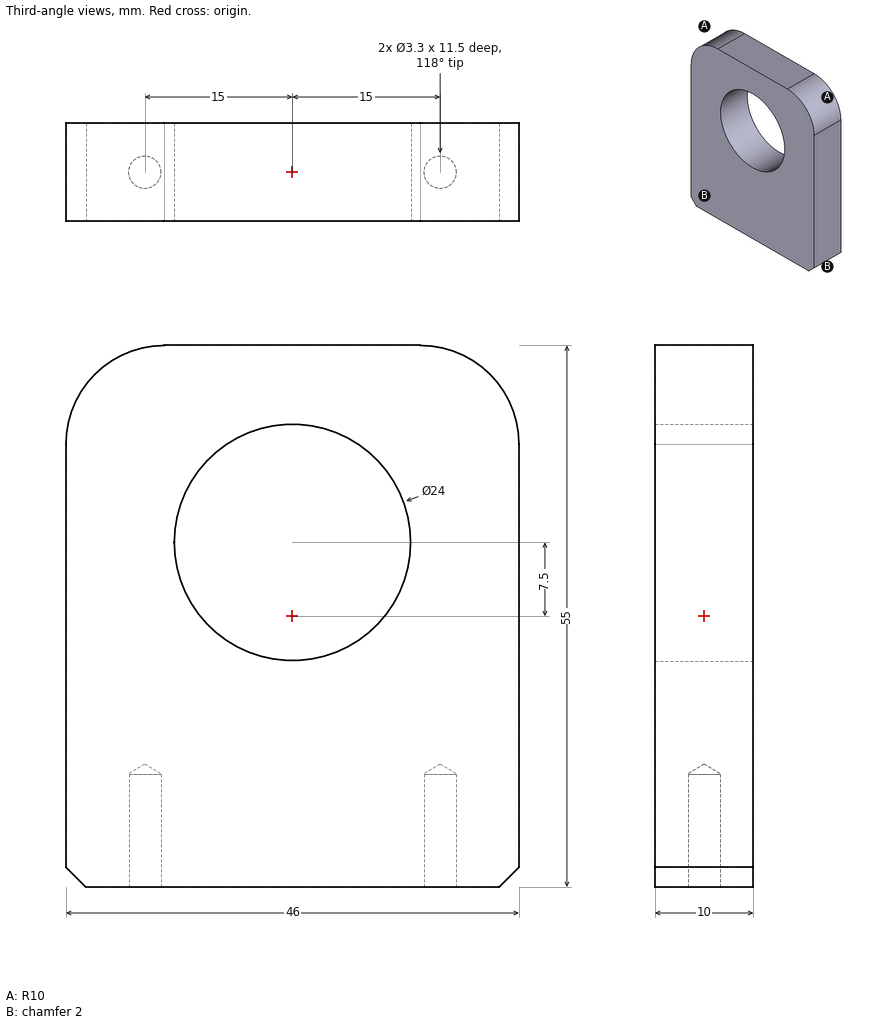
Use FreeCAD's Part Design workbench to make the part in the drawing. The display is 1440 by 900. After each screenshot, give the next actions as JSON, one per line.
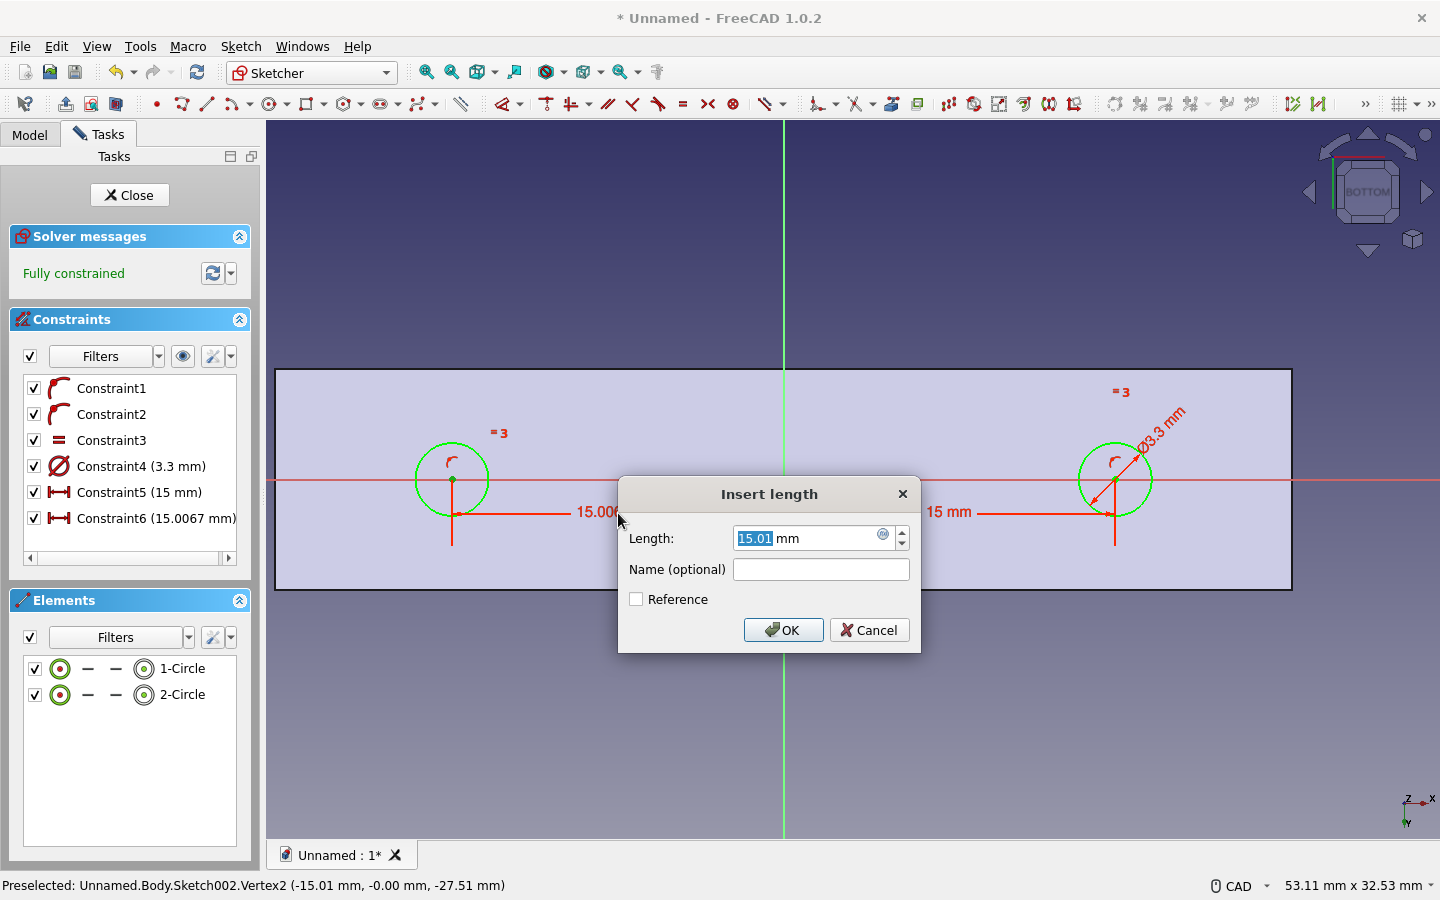
{"action": "type", "text": "15"}
{"action": "key", "text": "Return"}
{"action": "key", "text": "Escape"}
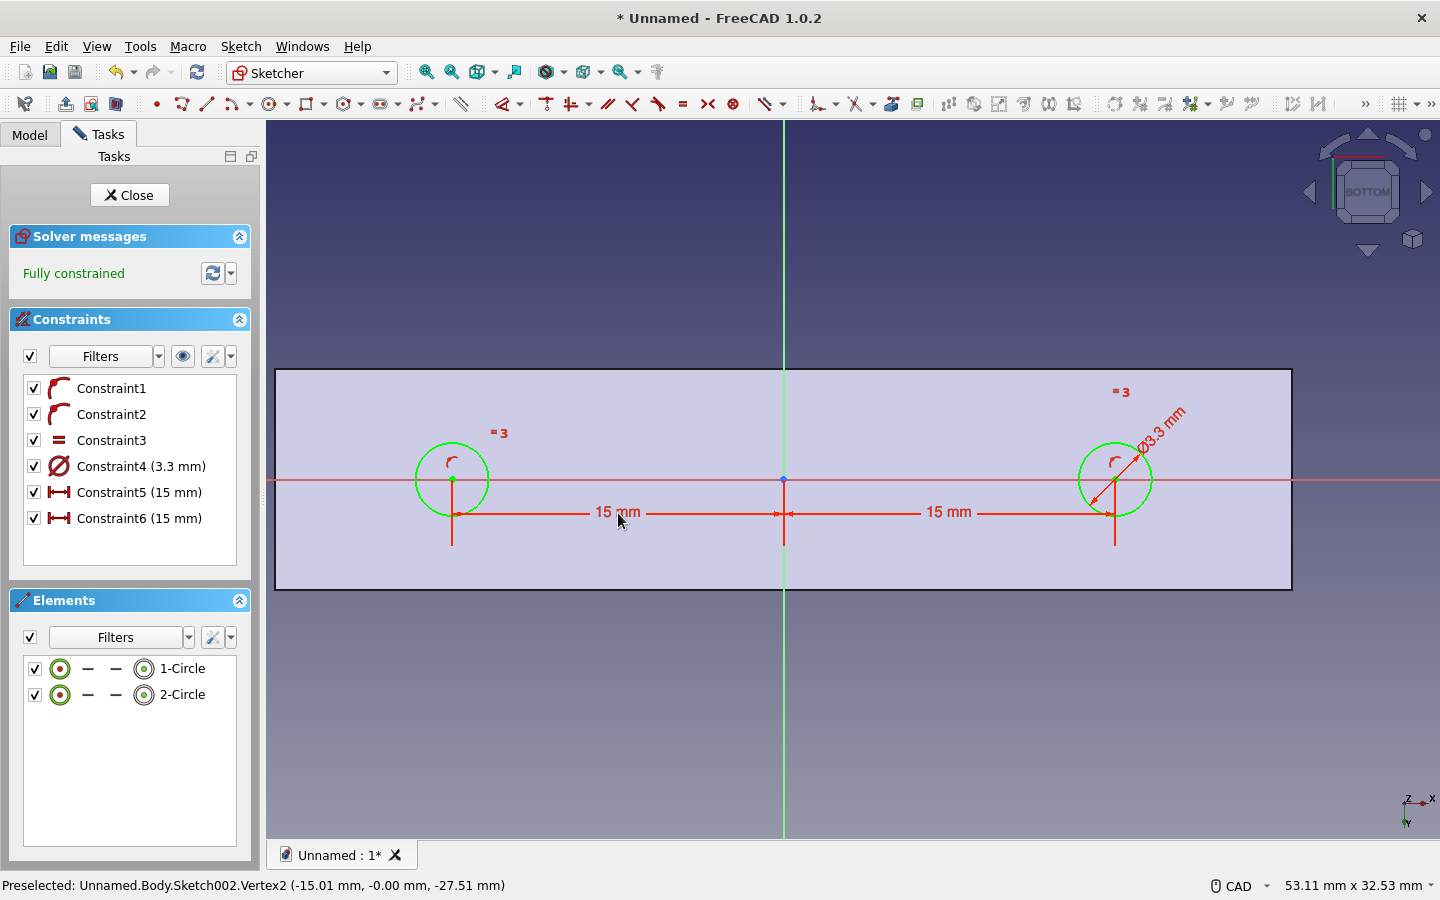
{"action": "left_click", "coordinate": [130, 195]}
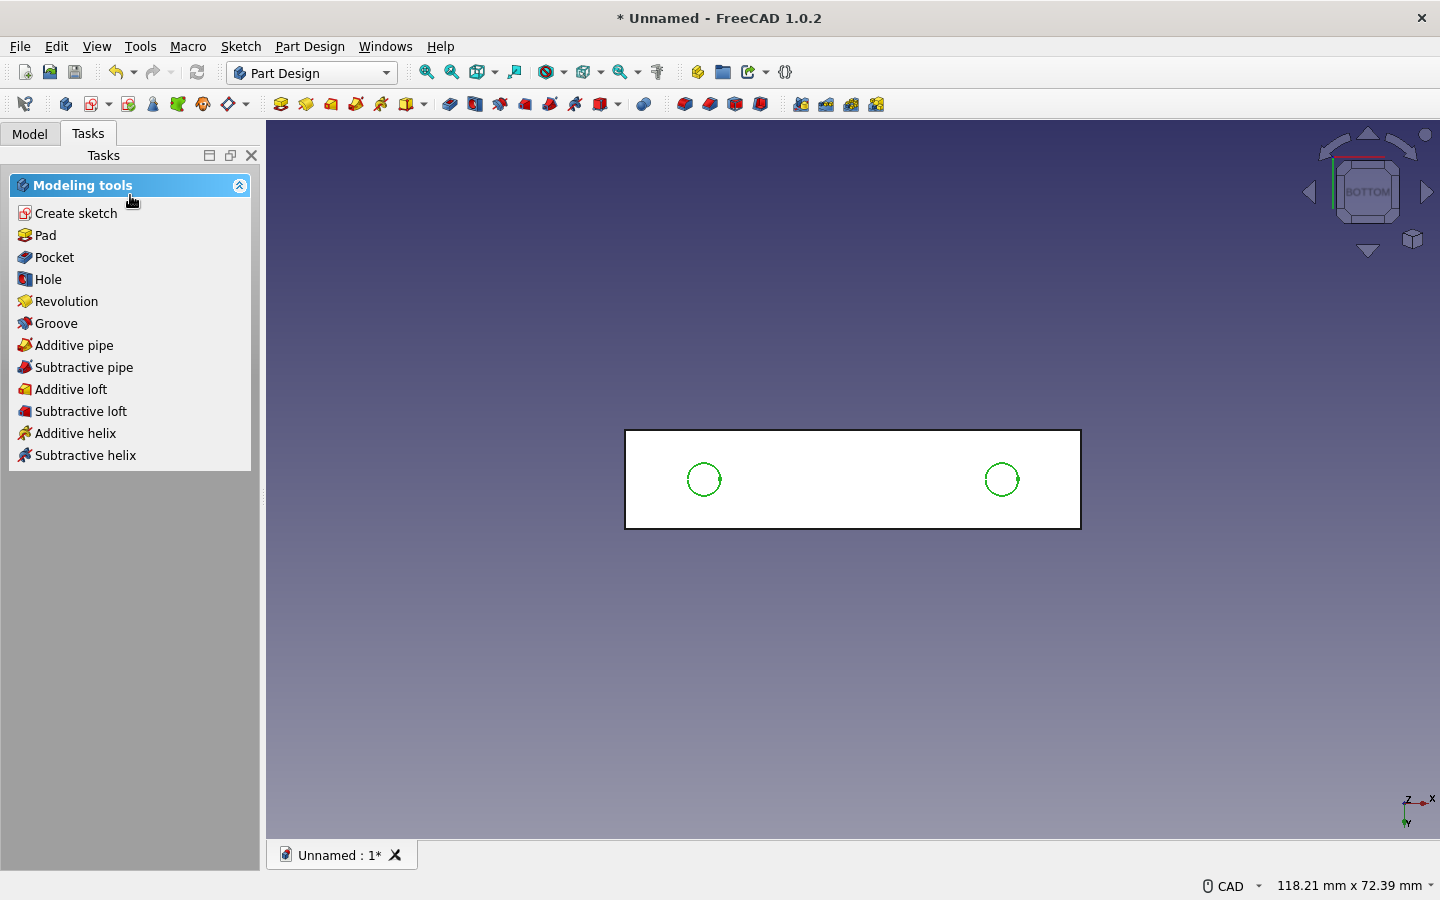
{"action": "left_click", "coordinate": [475, 104]}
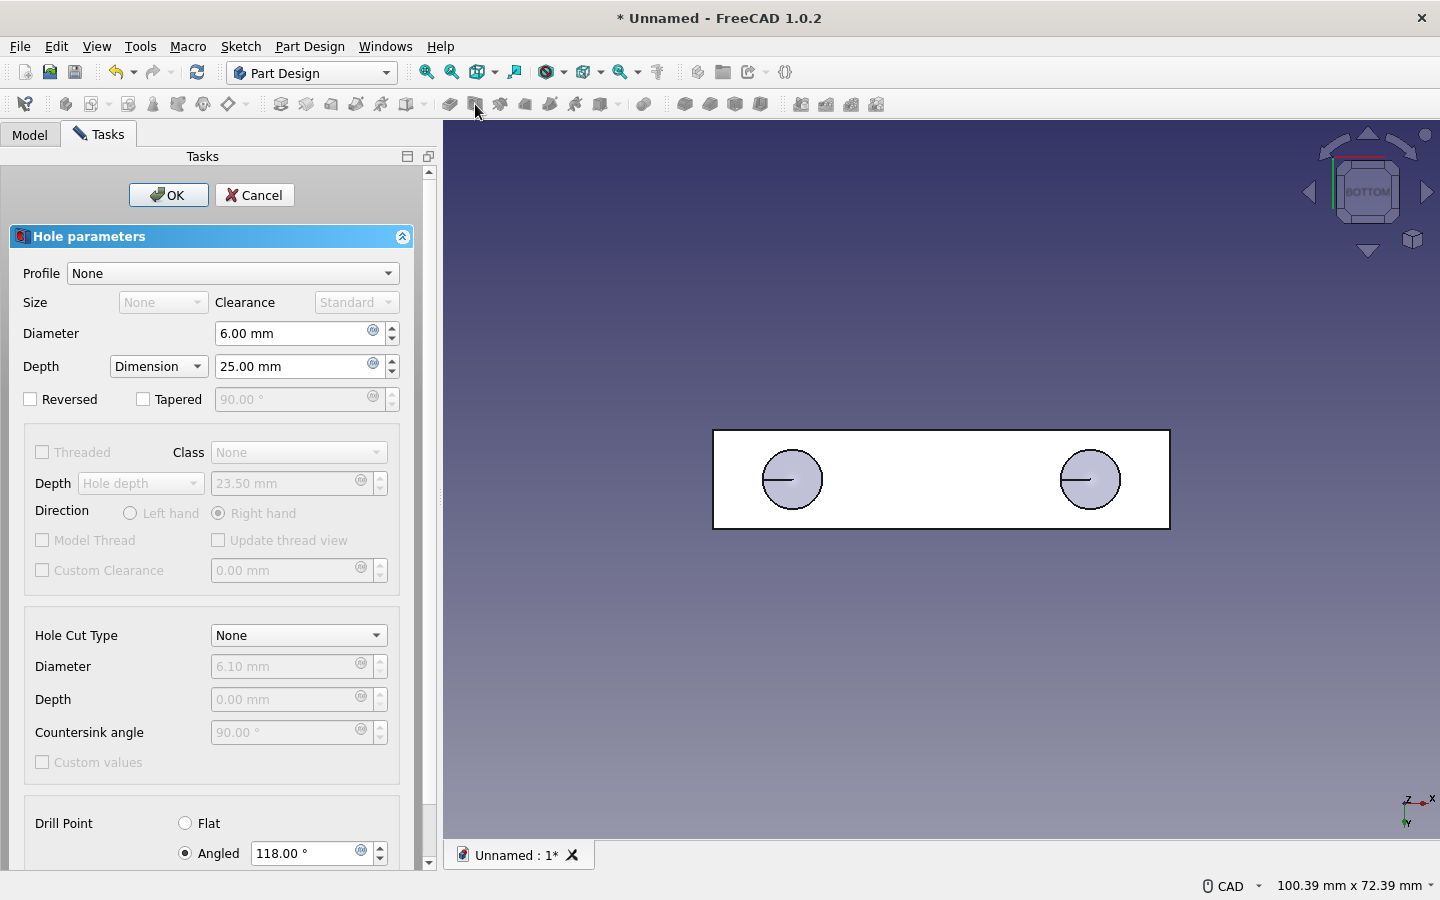
{"action": "triple_click", "coordinate": [300, 334]}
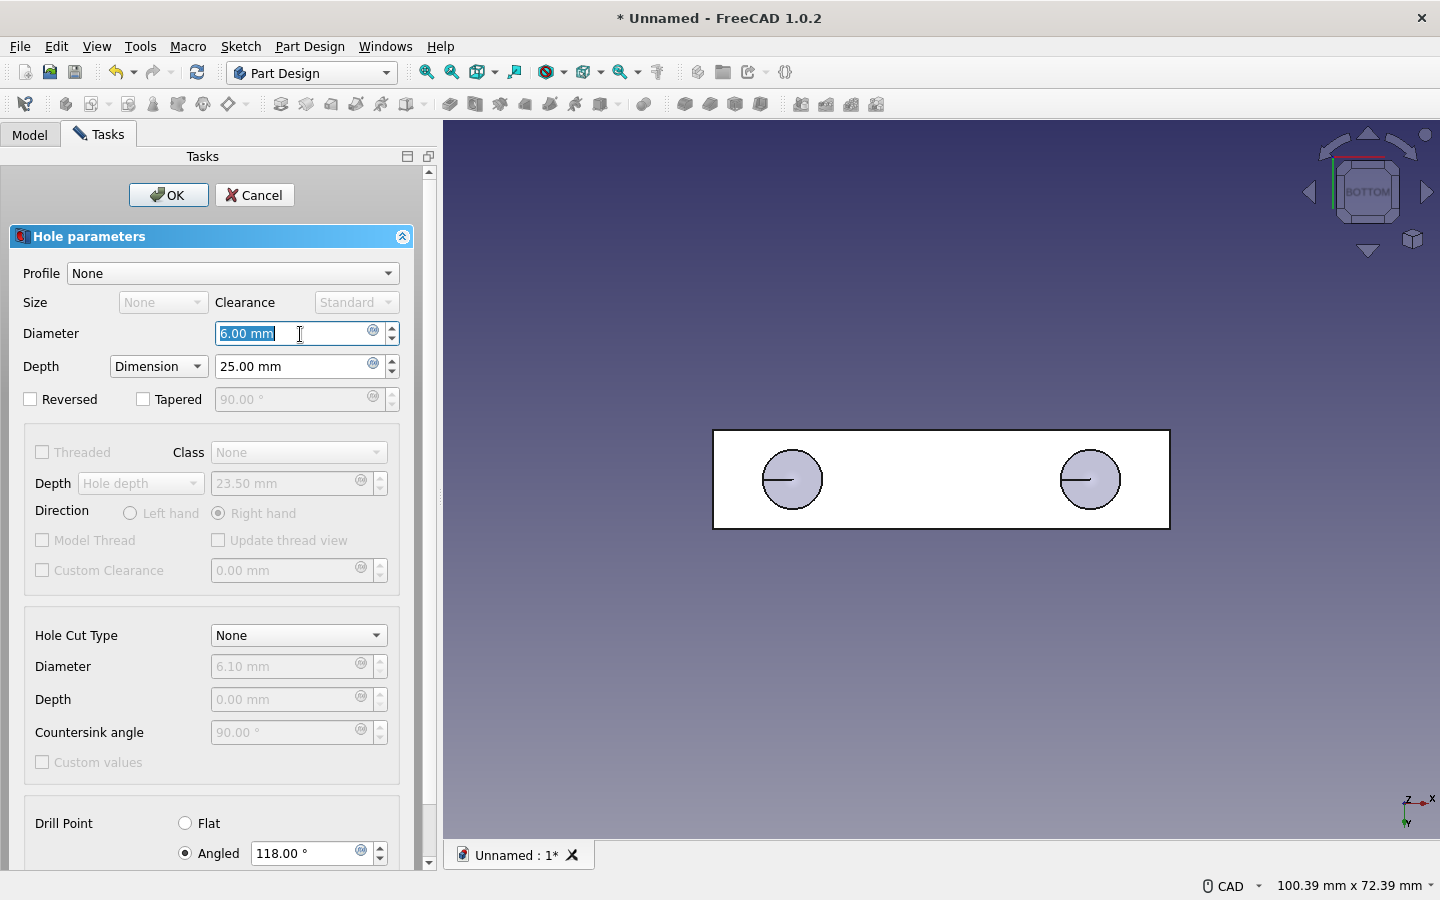
{"action": "type", "text": "3.3"}
{"action": "key", "text": "Tab"}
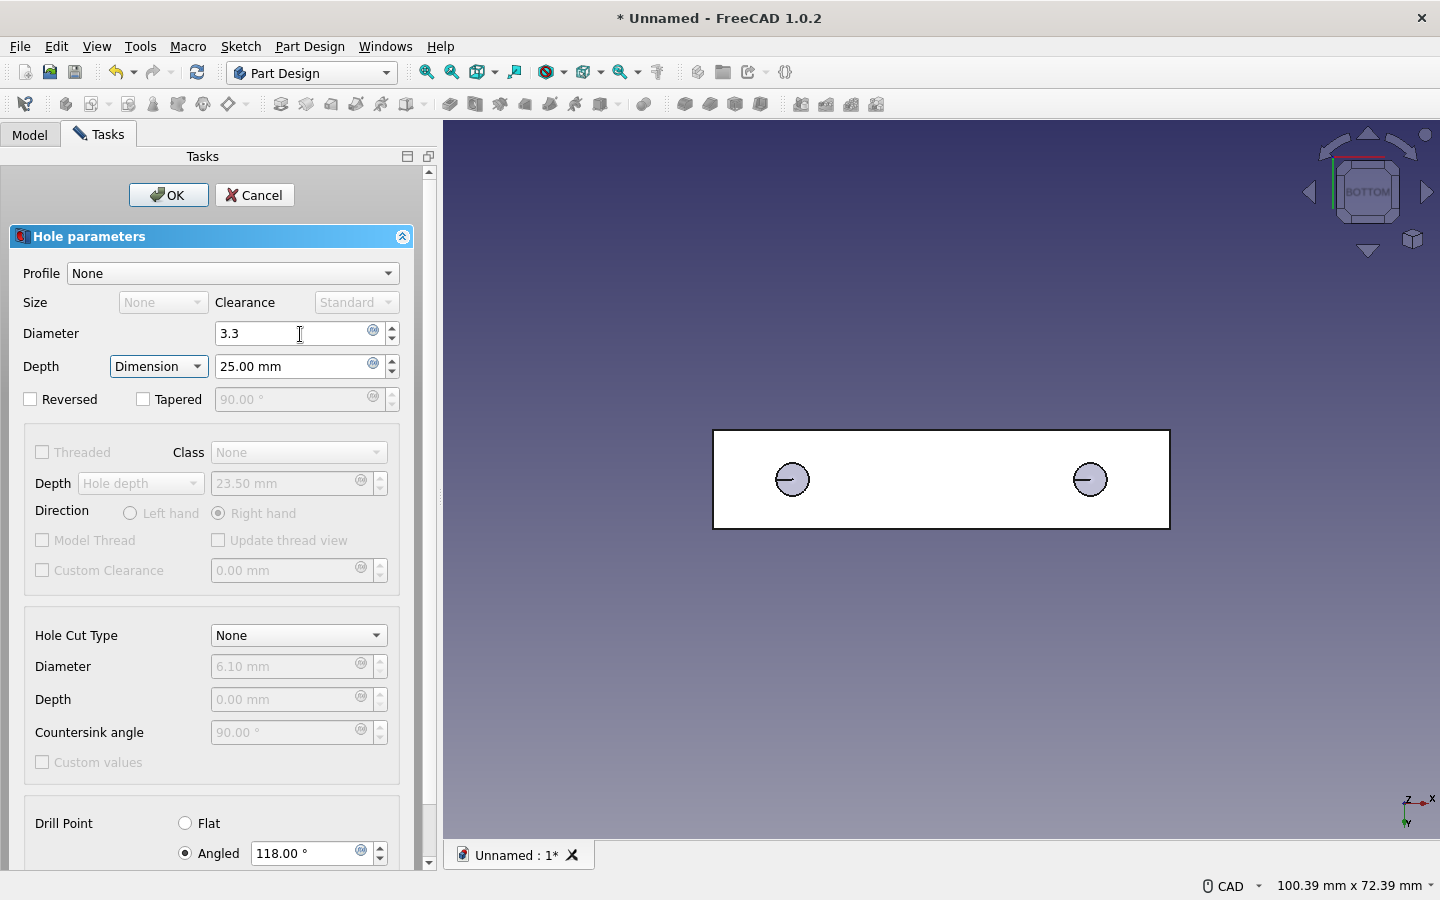
{"action": "triple_click", "coordinate": [300, 366]}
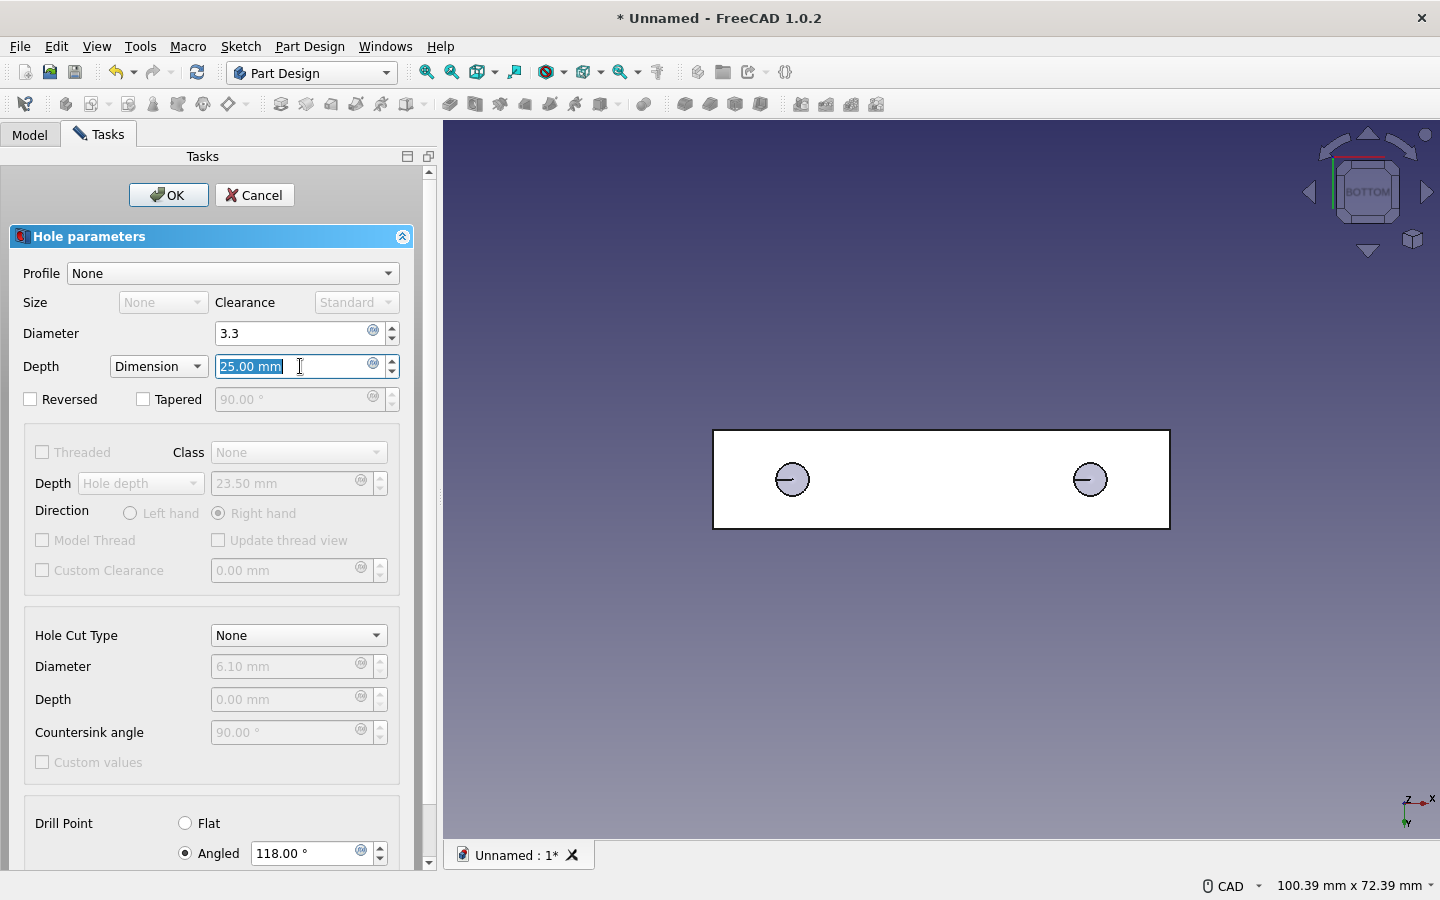
{"action": "type", "text": "11.5"}
{"action": "key", "text": "Tab"}